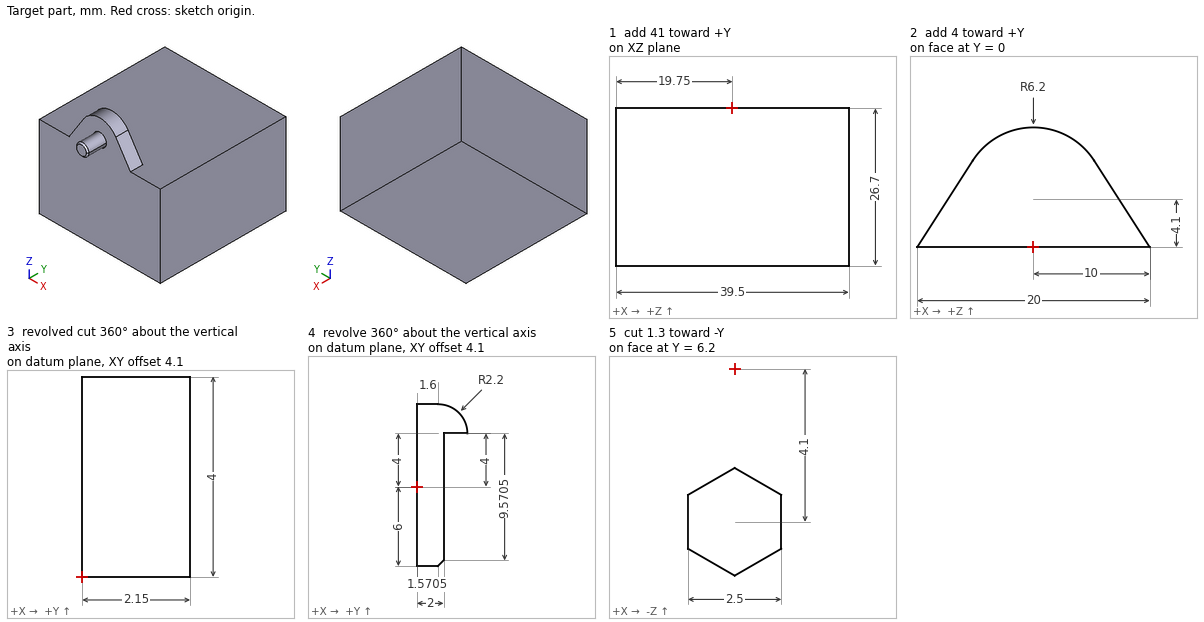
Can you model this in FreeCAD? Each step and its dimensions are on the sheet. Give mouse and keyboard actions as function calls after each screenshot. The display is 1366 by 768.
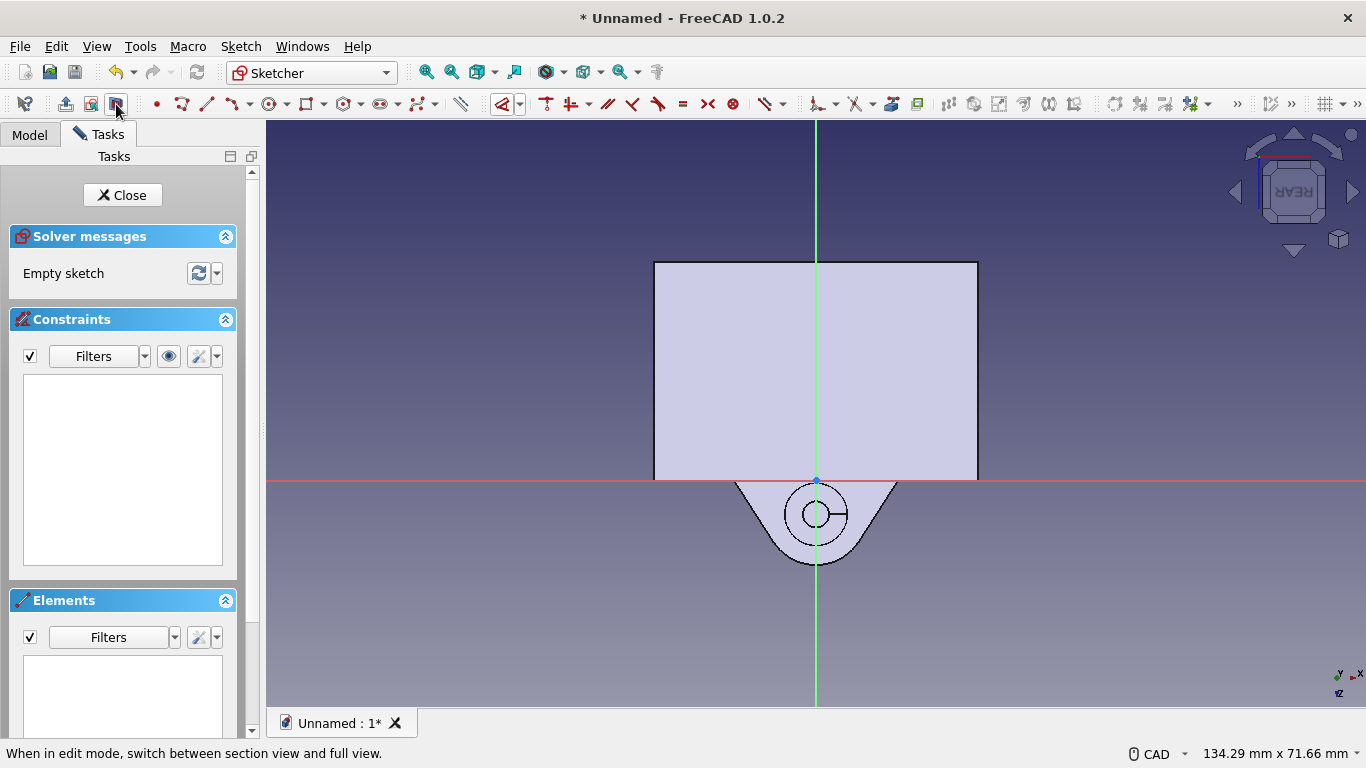
scroll(825, 515, up, 11)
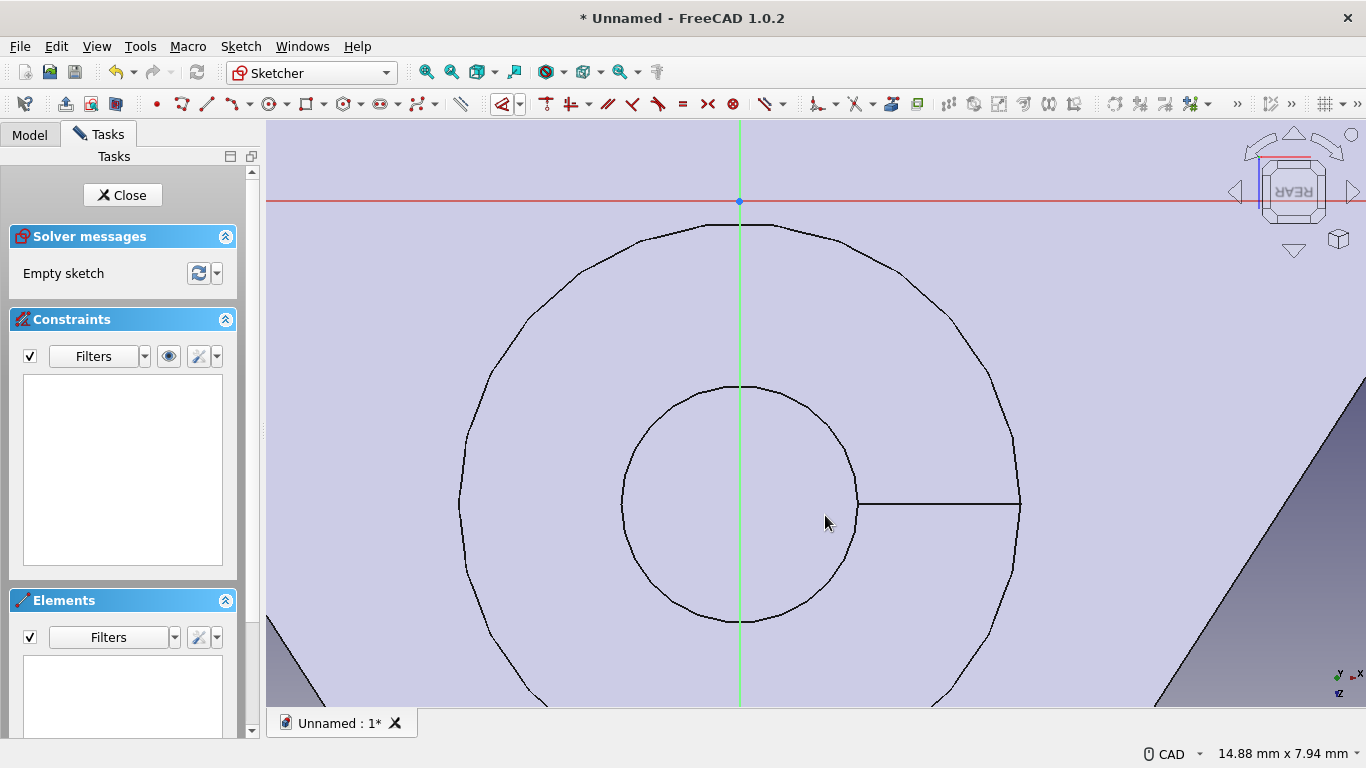
key(g)
key(p)
key(6)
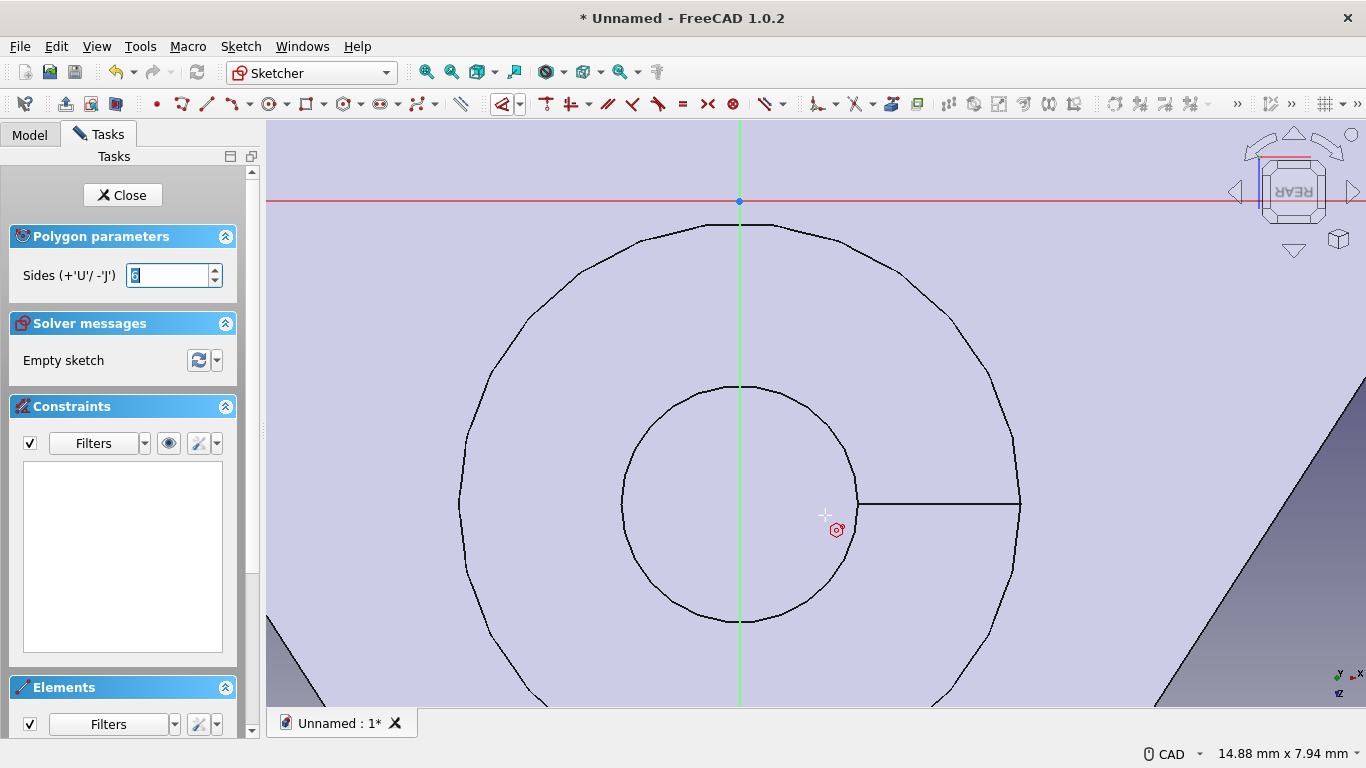
click(740, 504)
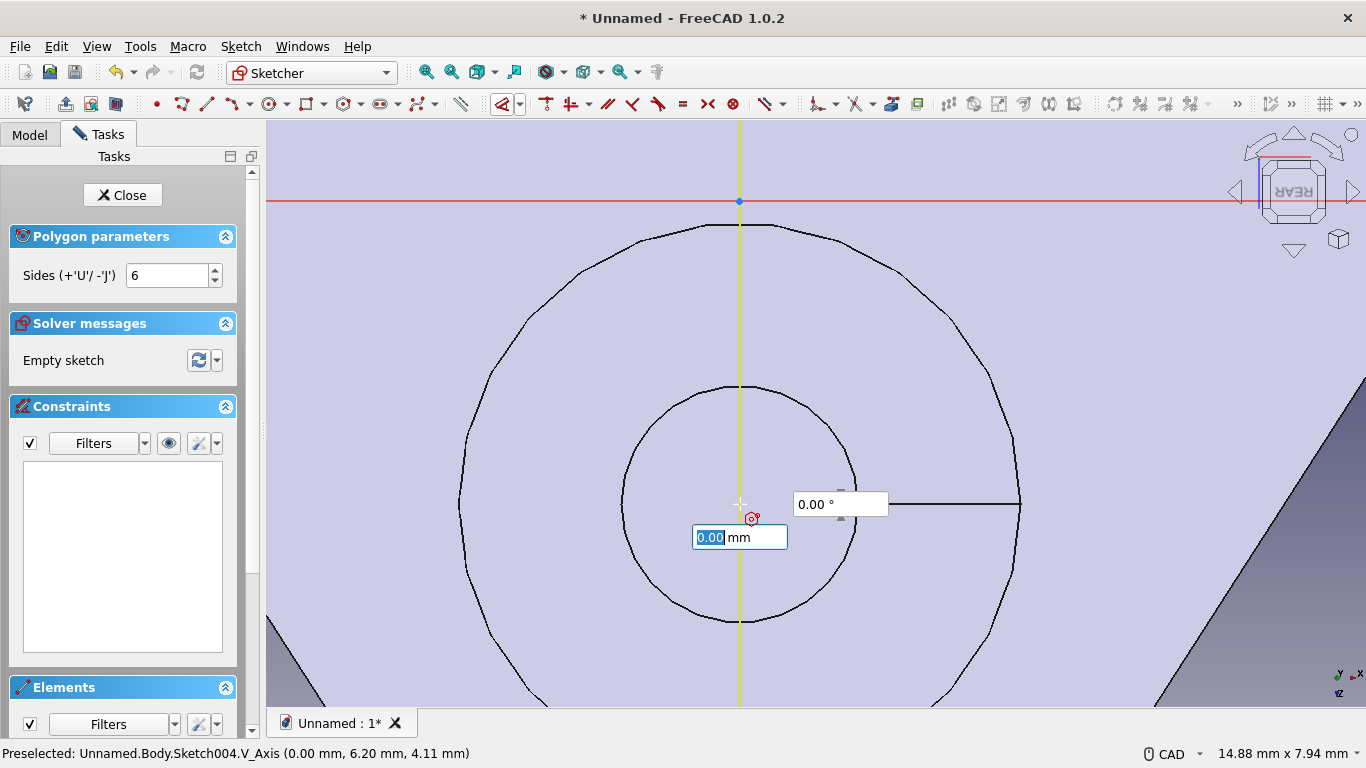
click(740, 611)
right_click(740, 611)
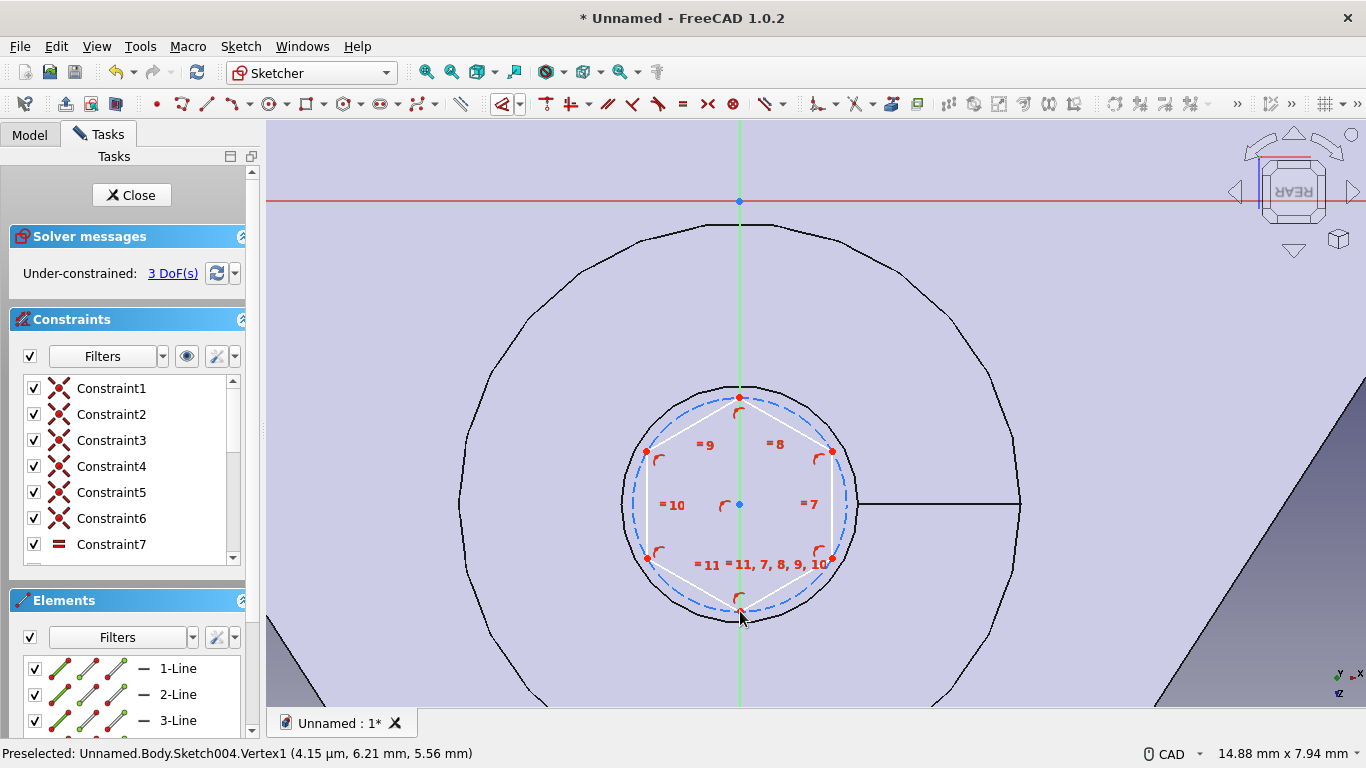
click(832, 526)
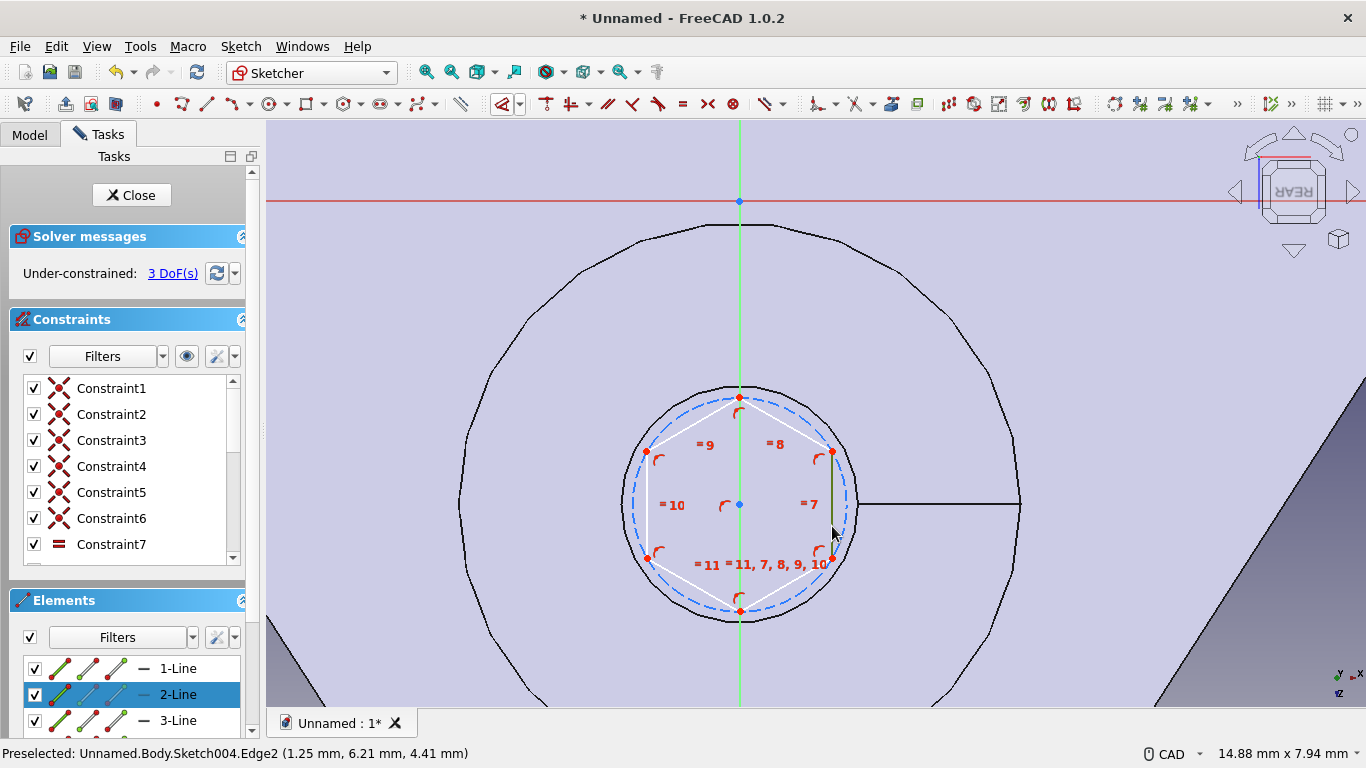
click(588, 104)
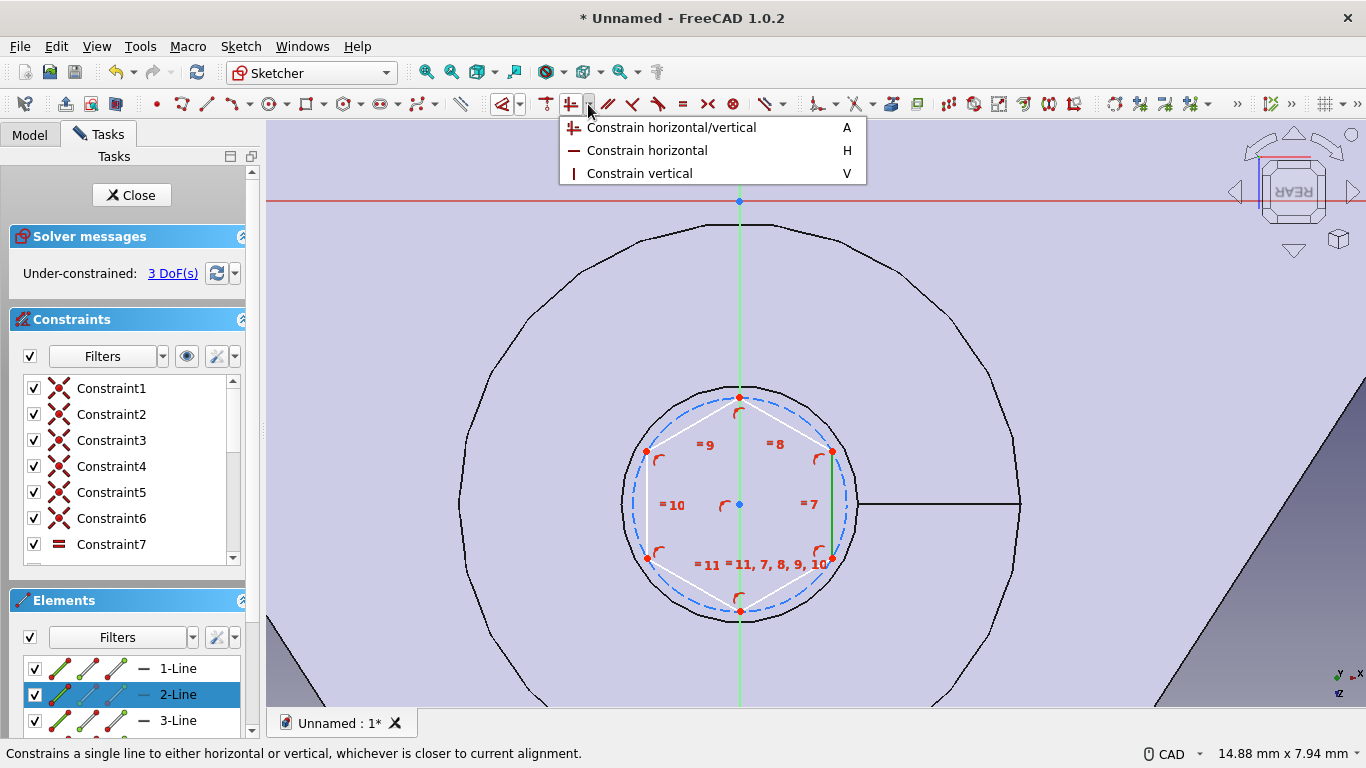
click(713, 174)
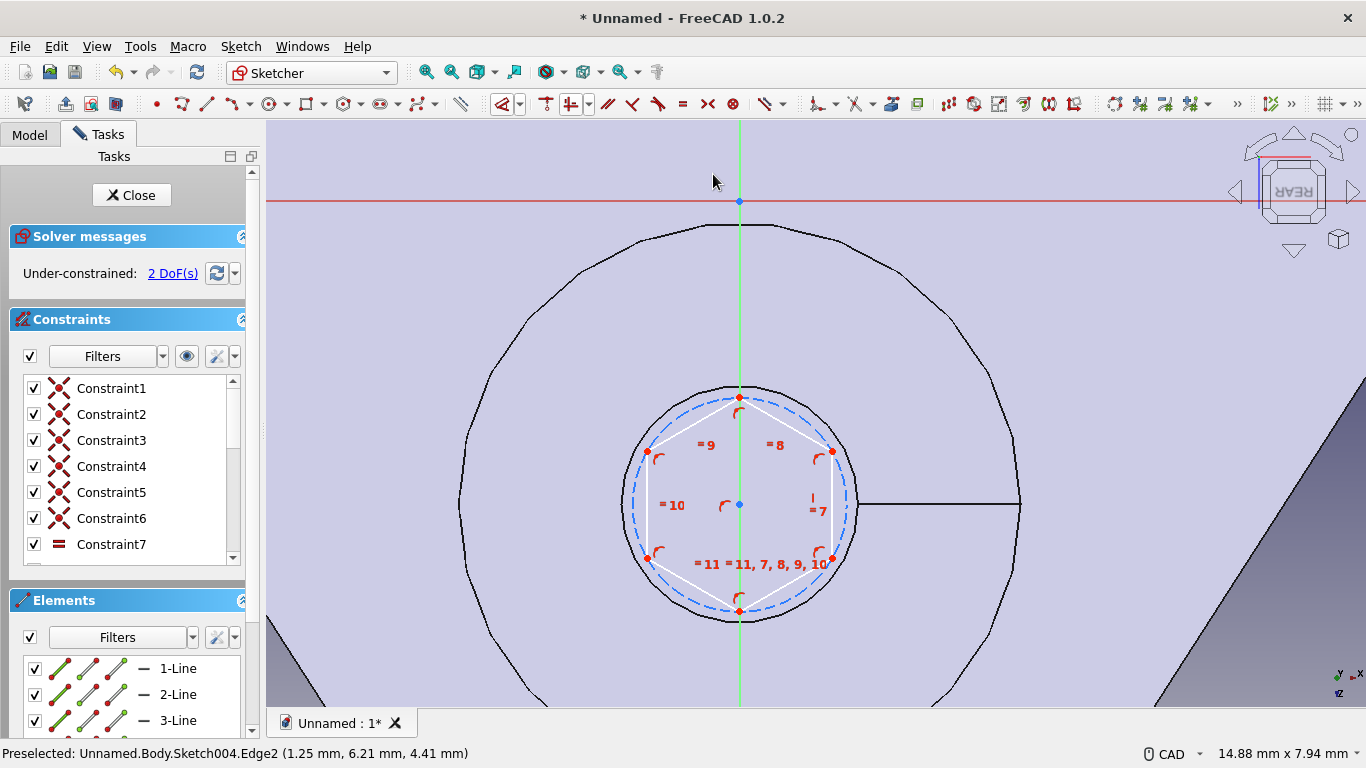
click(647, 451)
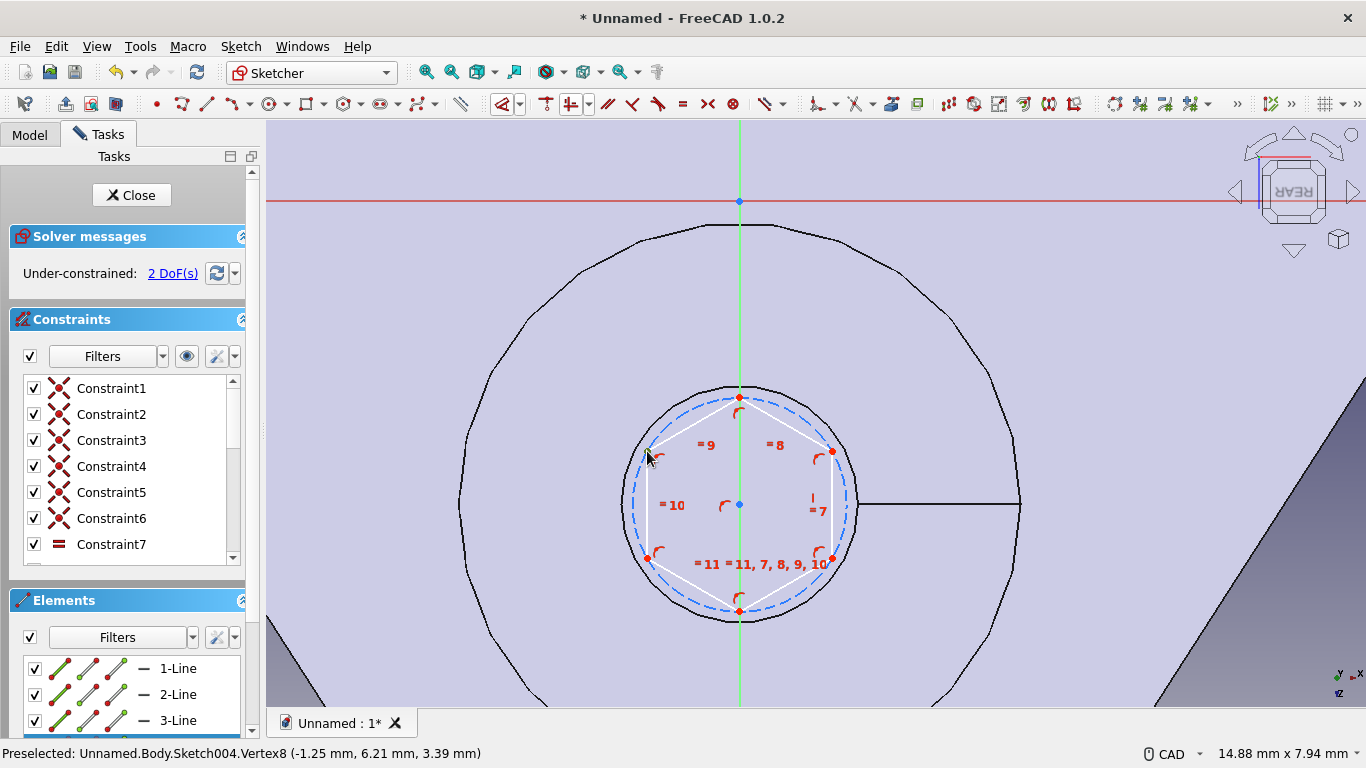
click(832, 558)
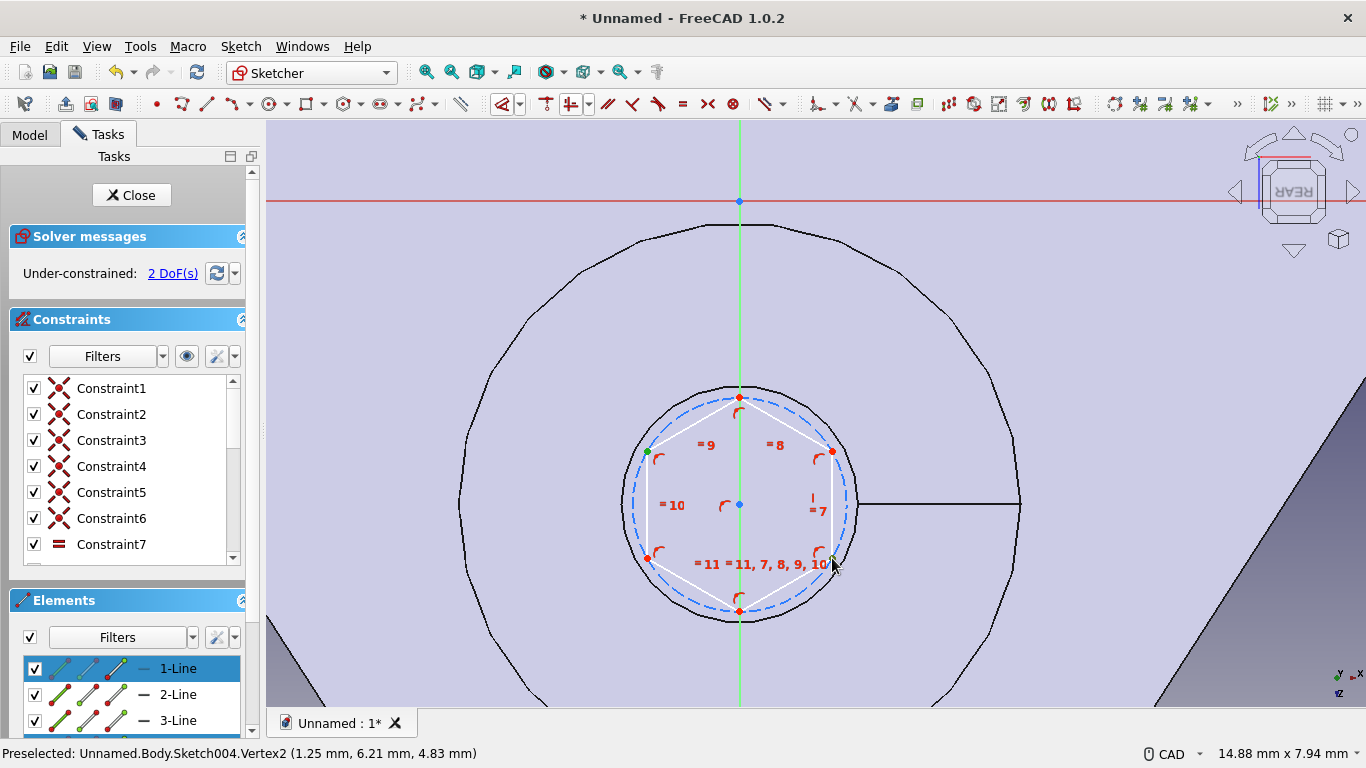
key(l)